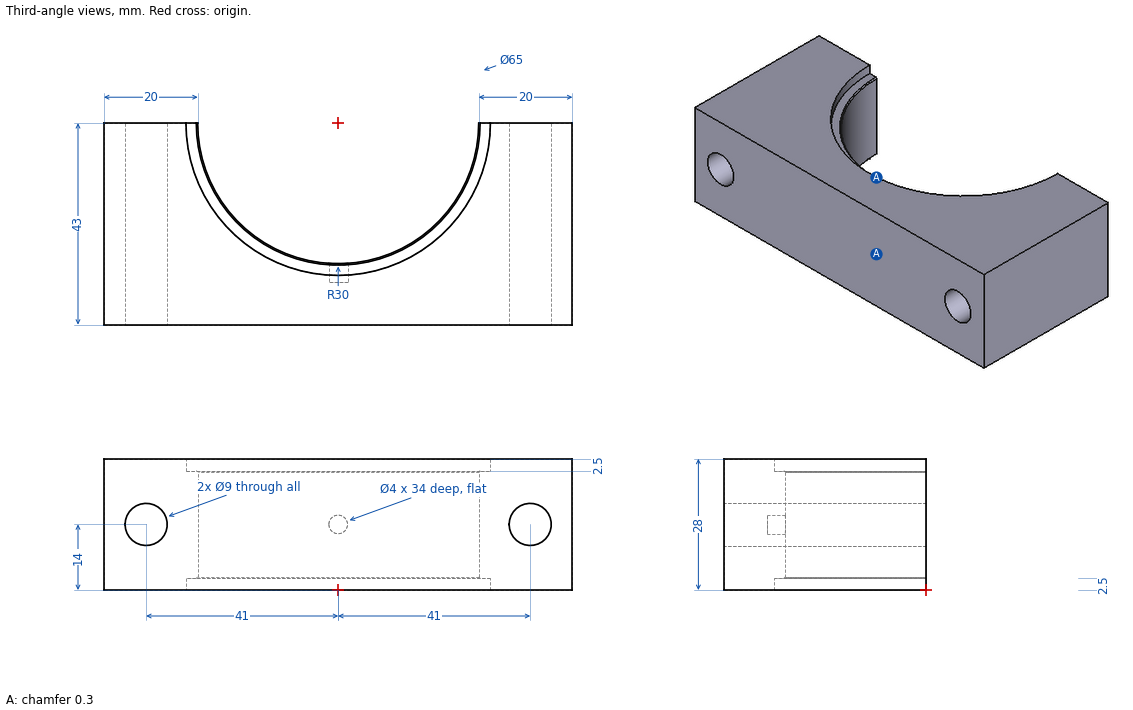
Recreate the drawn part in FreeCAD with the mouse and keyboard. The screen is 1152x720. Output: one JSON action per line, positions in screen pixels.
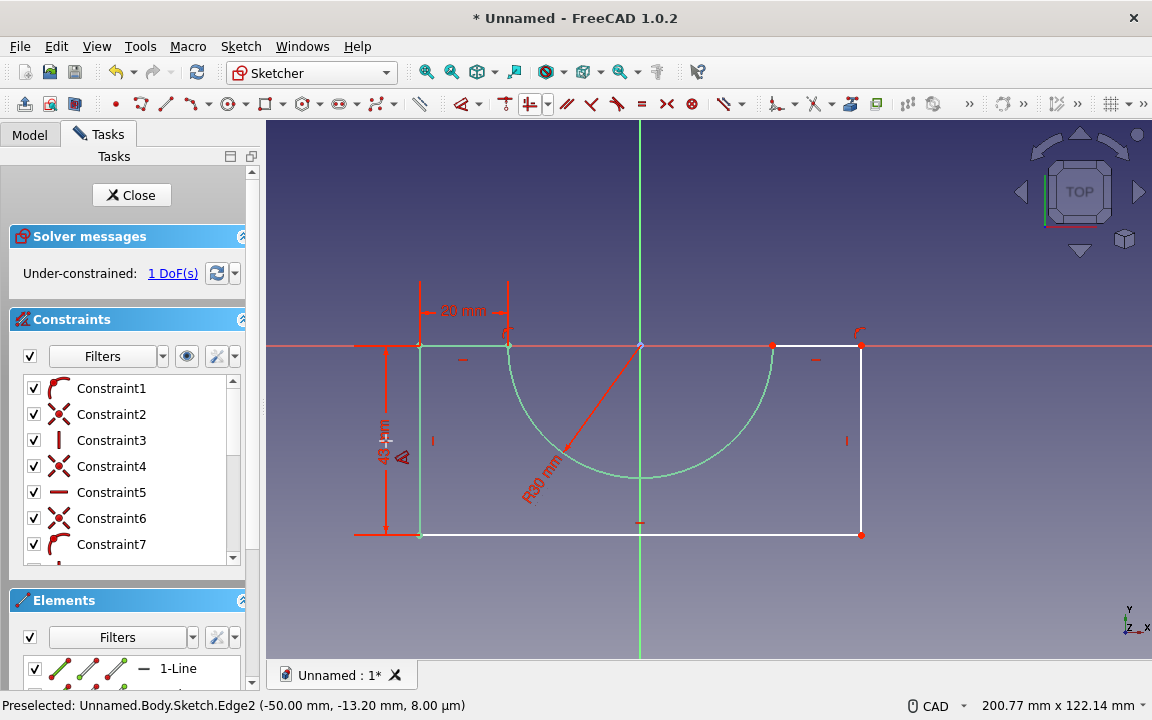
{"action": "left_click", "coordinate": [835, 346]}
{"action": "left_click", "coordinate": [817, 312]}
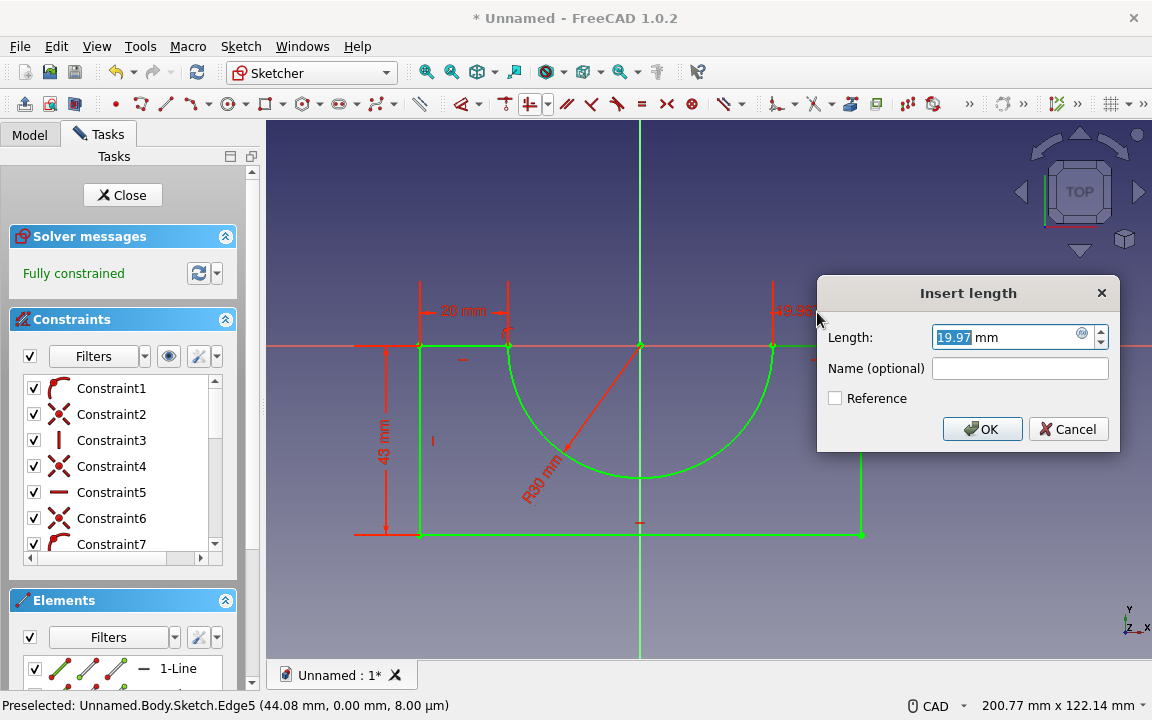
{"action": "type", "text": "20"}
{"action": "key", "text": "Return"}
{"action": "key", "text": "Escape"}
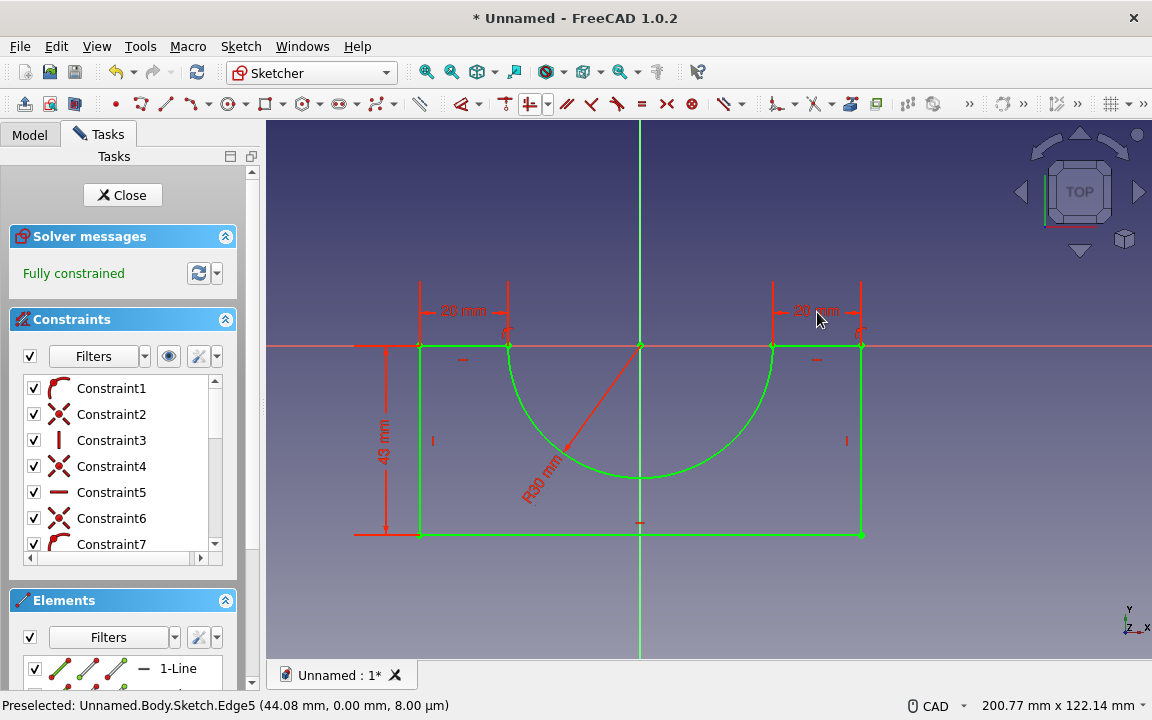
{"action": "left_click", "coordinate": [123, 195]}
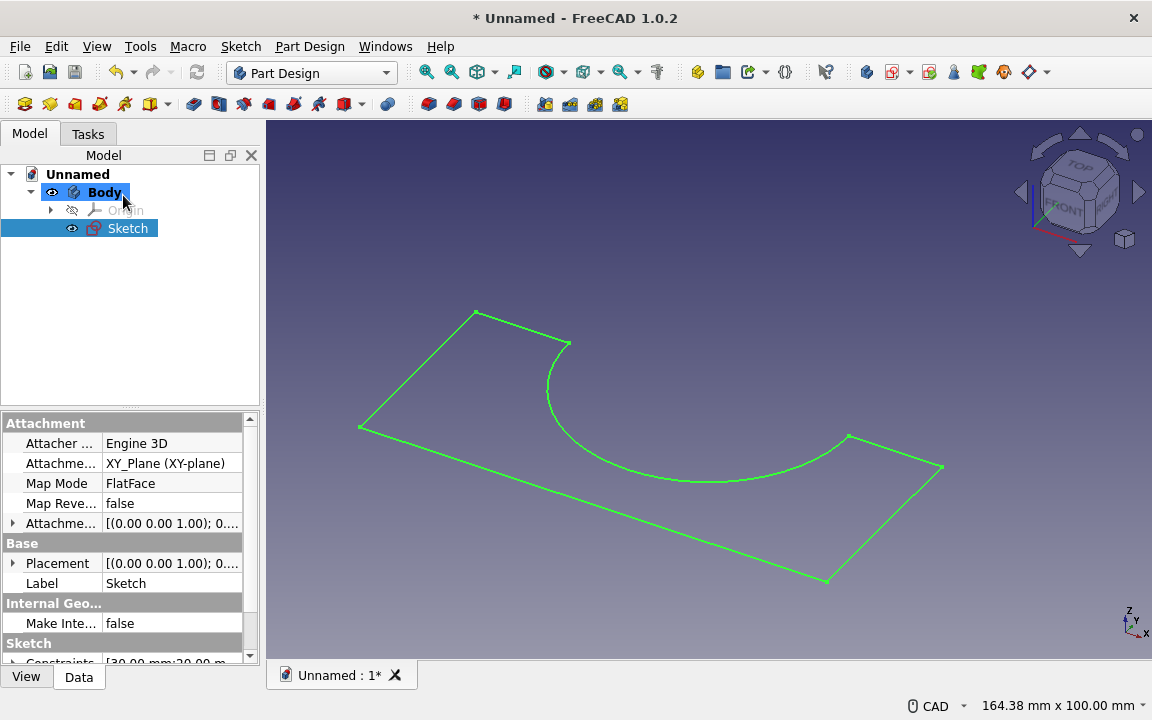
{"action": "left_click", "coordinate": [25, 104]}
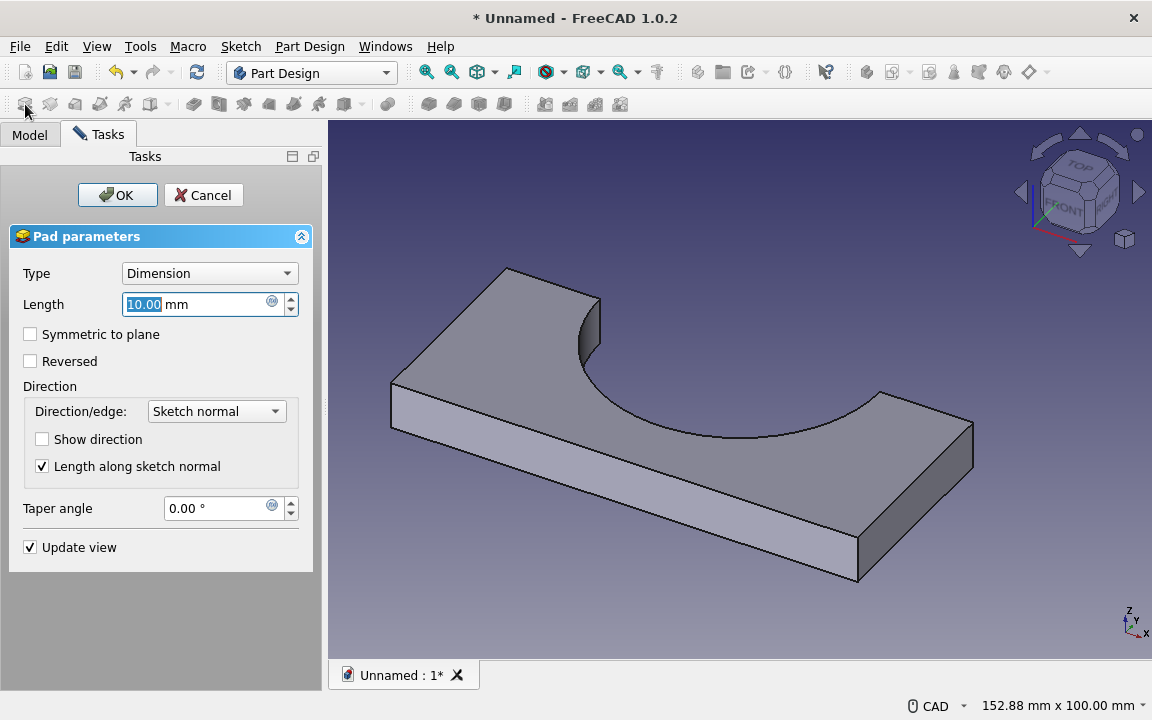
{"action": "type", "text": "28"}
{"action": "key", "text": "Tab"}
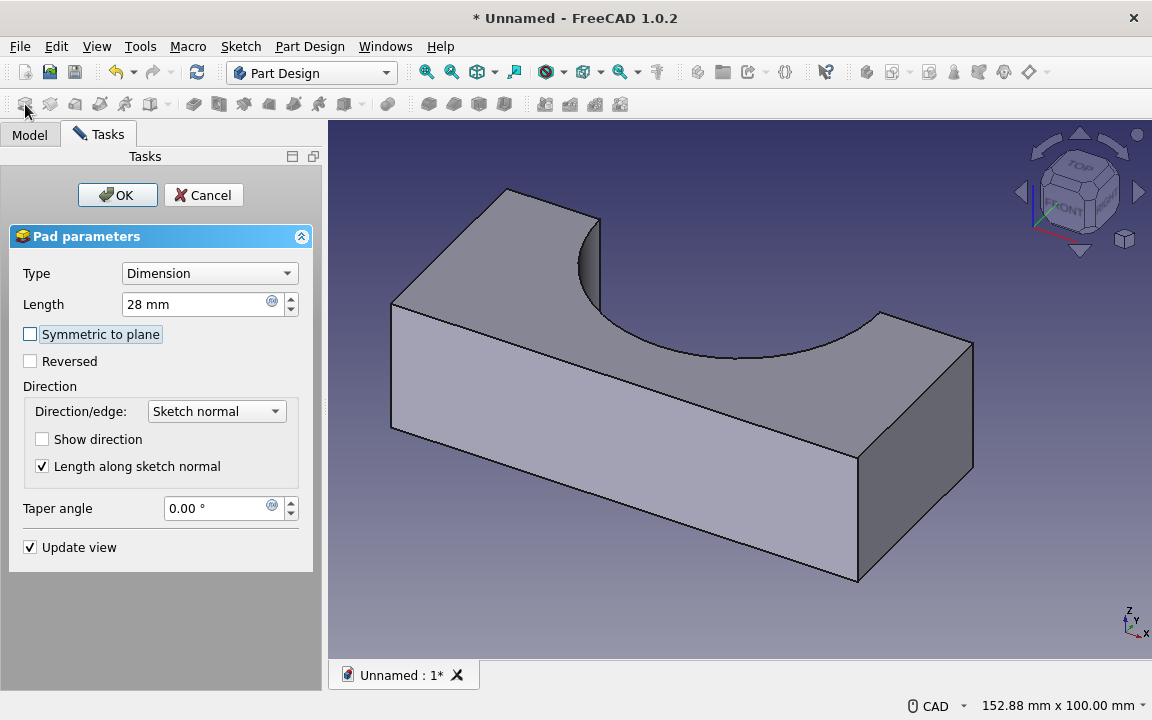
{"action": "left_click", "coordinate": [118, 195]}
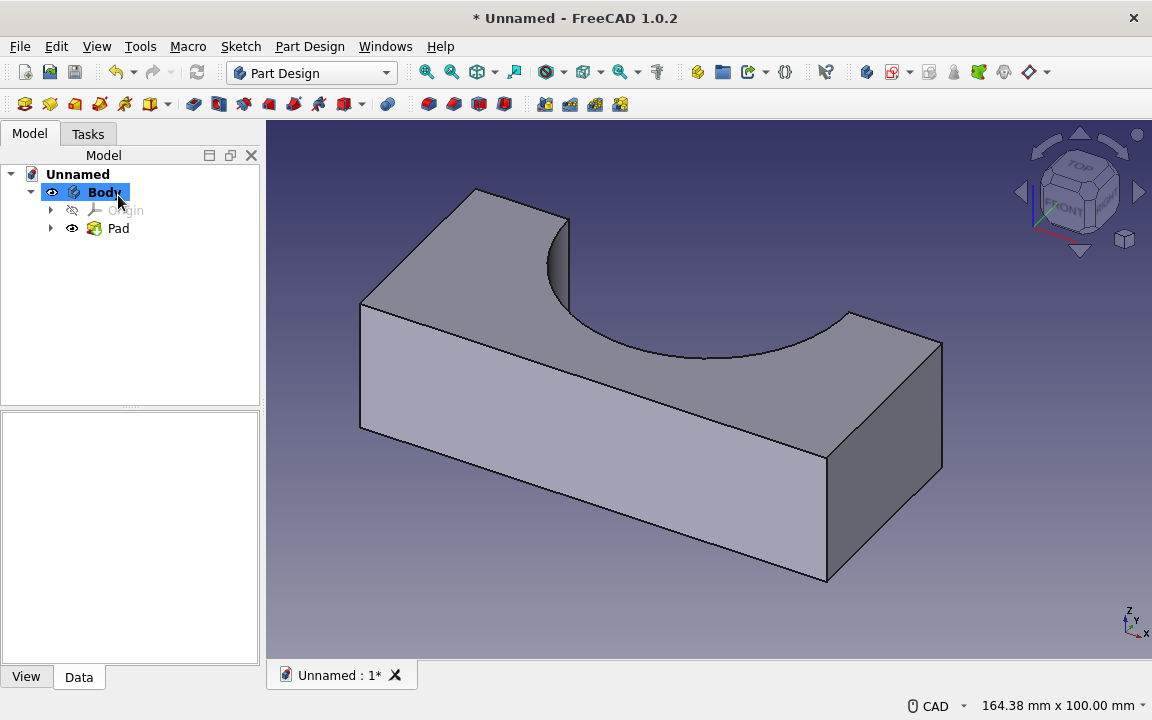
{"action": "left_click", "coordinate": [501, 295]}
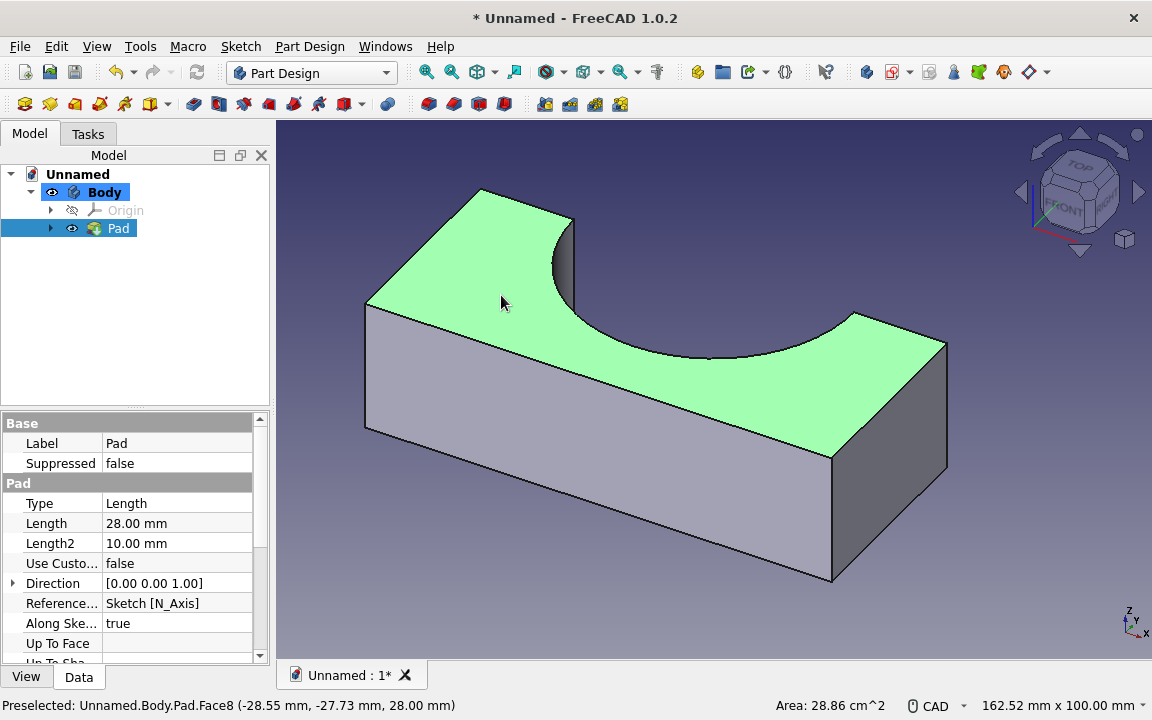
{"action": "left_click", "coordinate": [892, 72]}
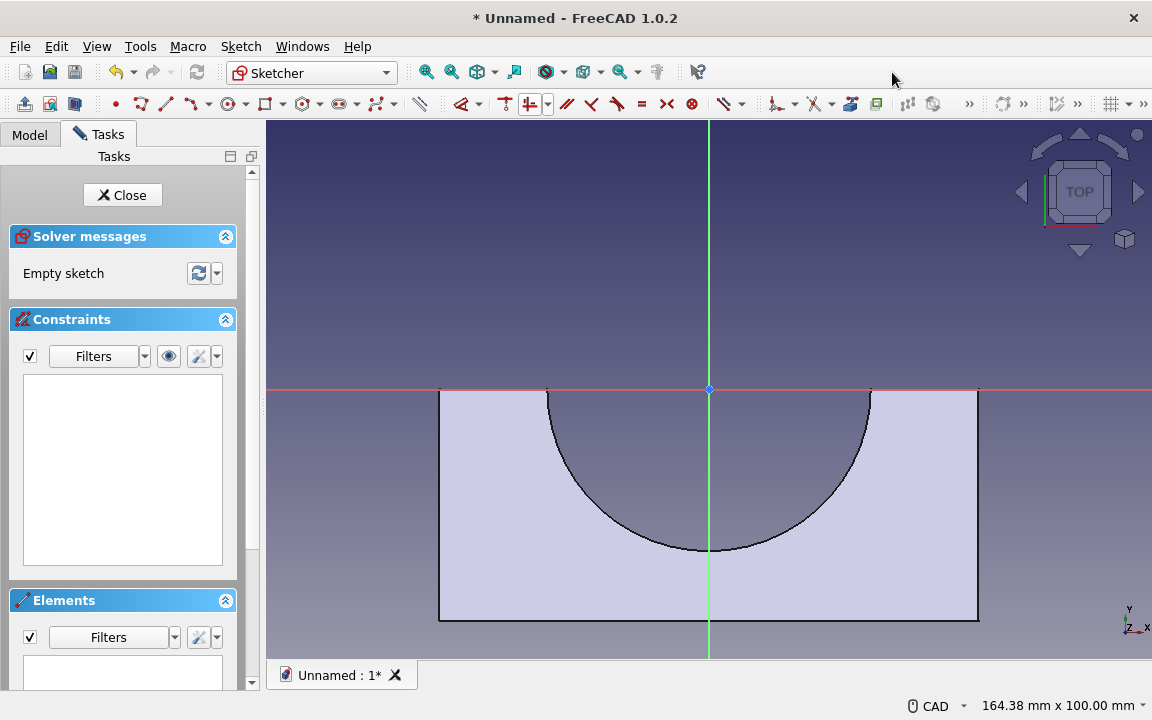
{"action": "left_click", "coordinate": [228, 104]}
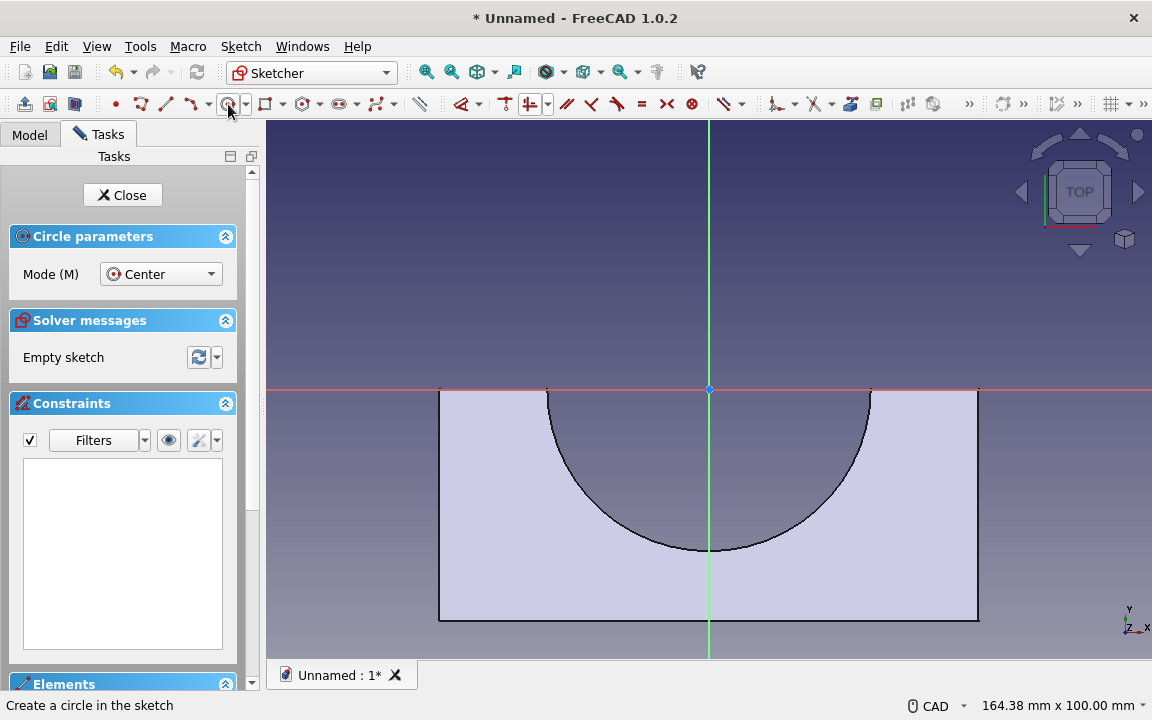
{"action": "left_click", "coordinate": [709, 390]}
{"action": "left_click", "coordinate": [833, 266]}
{"action": "key", "text": "Escape"}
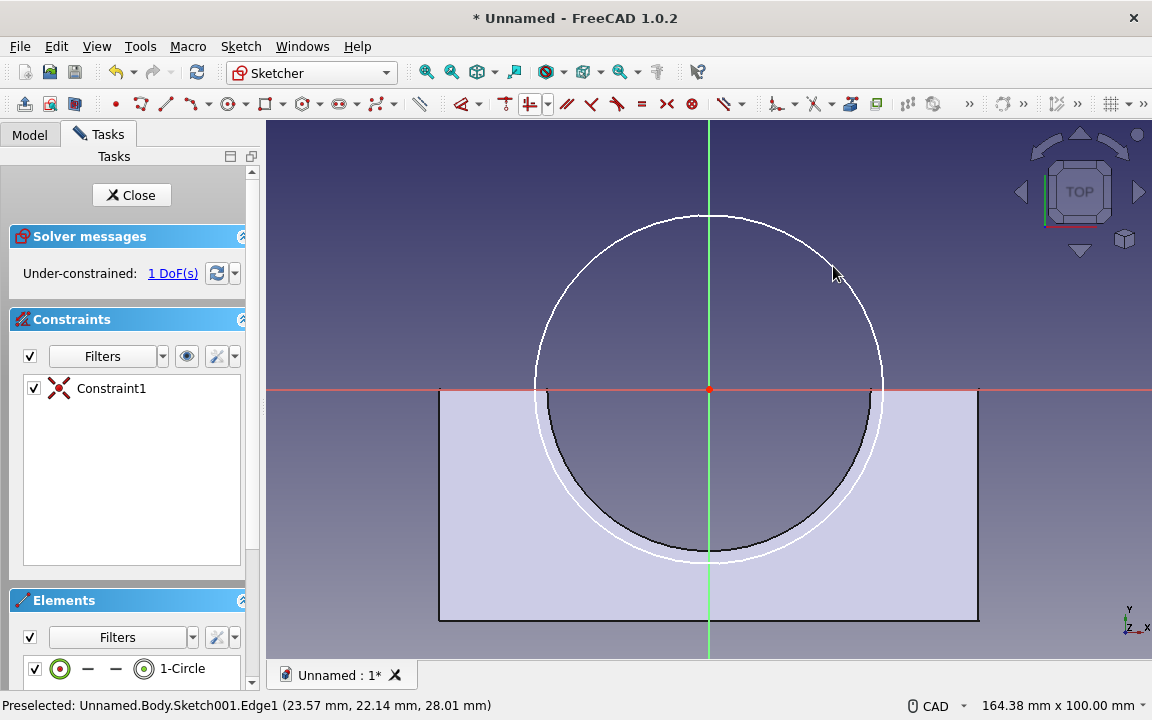
{"action": "left_click", "coordinate": [460, 104]}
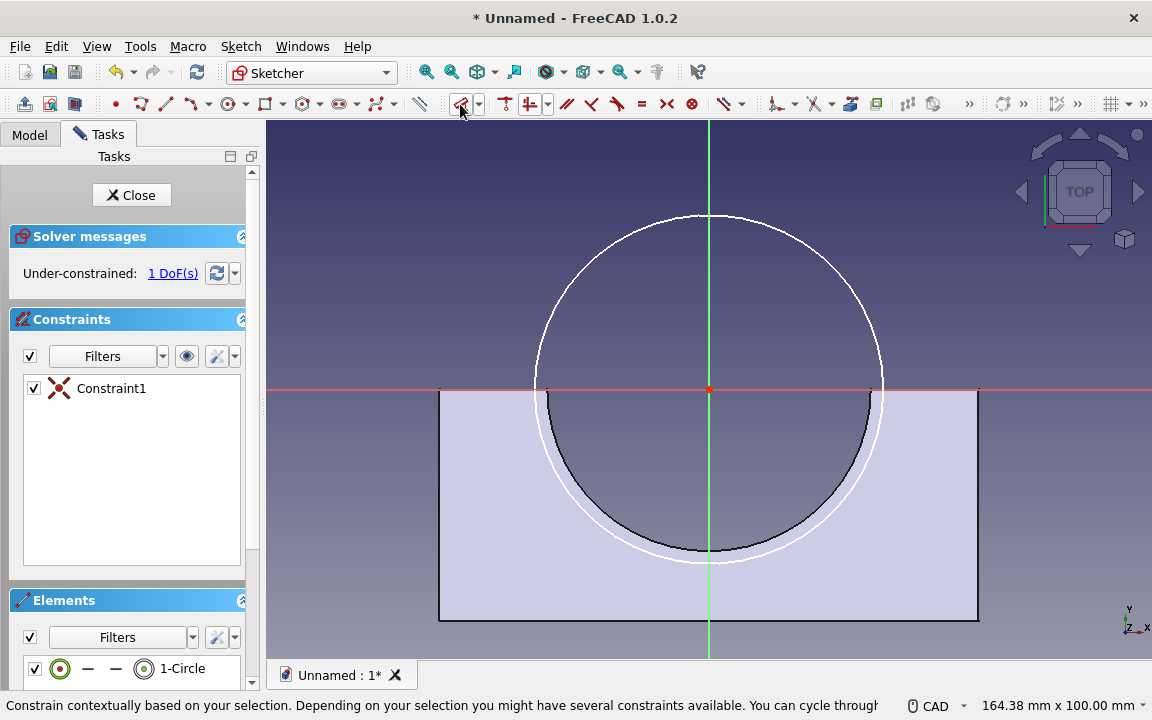
{"action": "left_click", "coordinate": [832, 266]}
{"action": "left_click", "coordinate": [855, 243]}